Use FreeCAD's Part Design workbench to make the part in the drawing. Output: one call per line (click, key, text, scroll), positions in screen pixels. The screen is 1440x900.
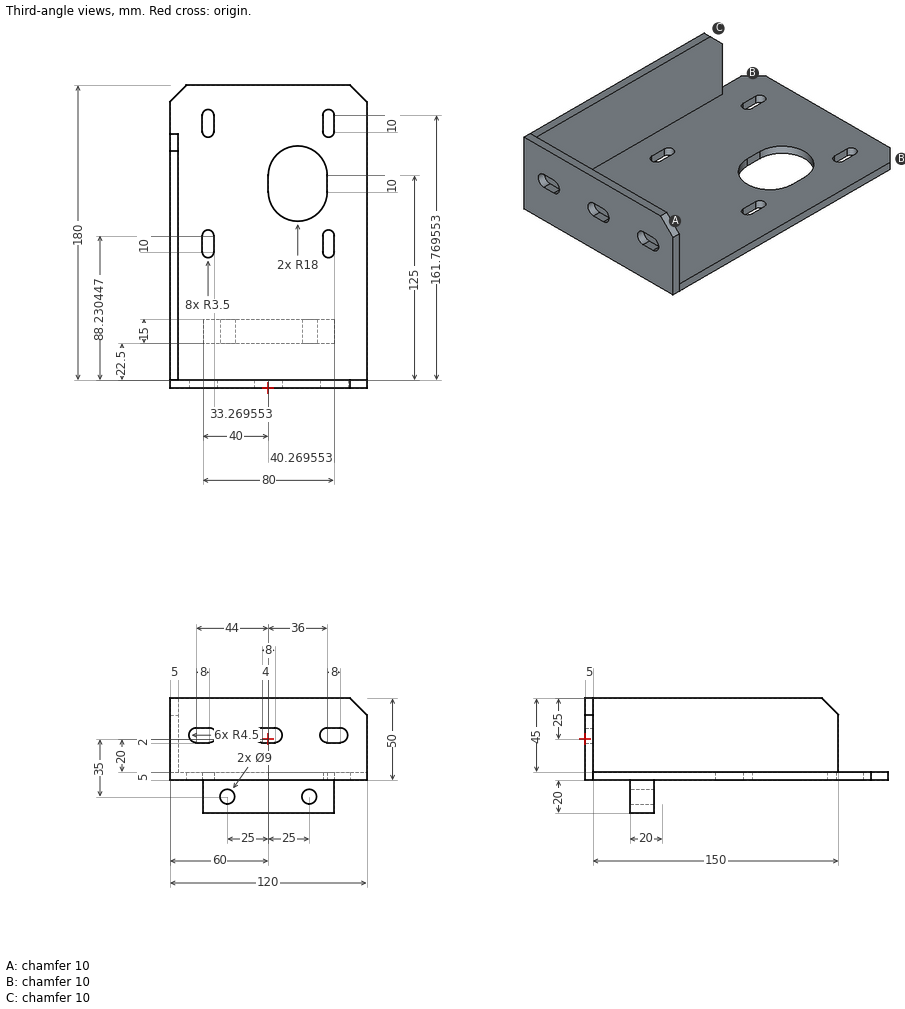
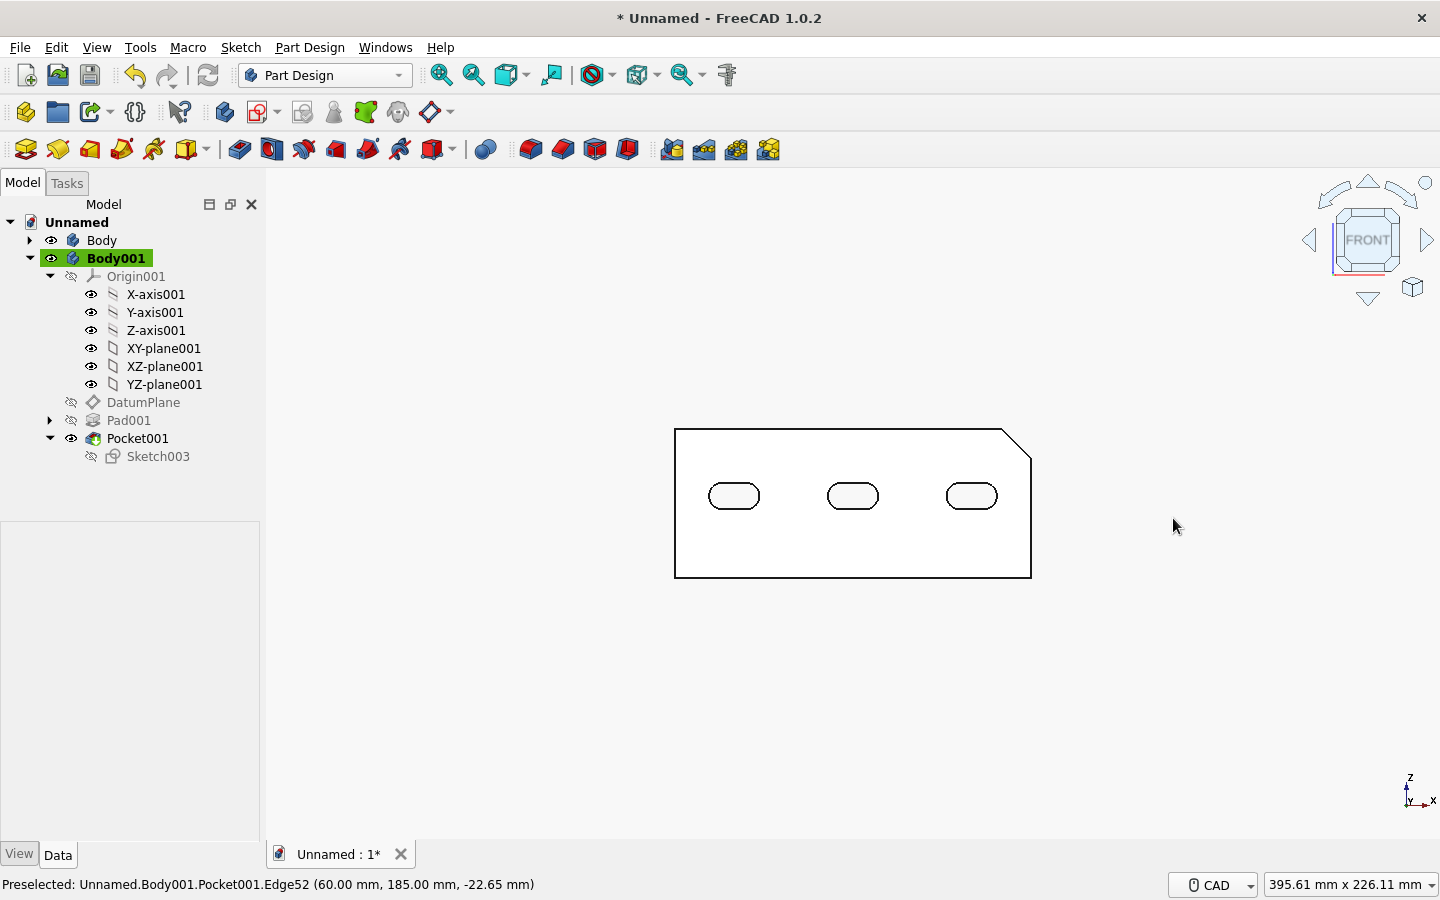
key(v)
key(f)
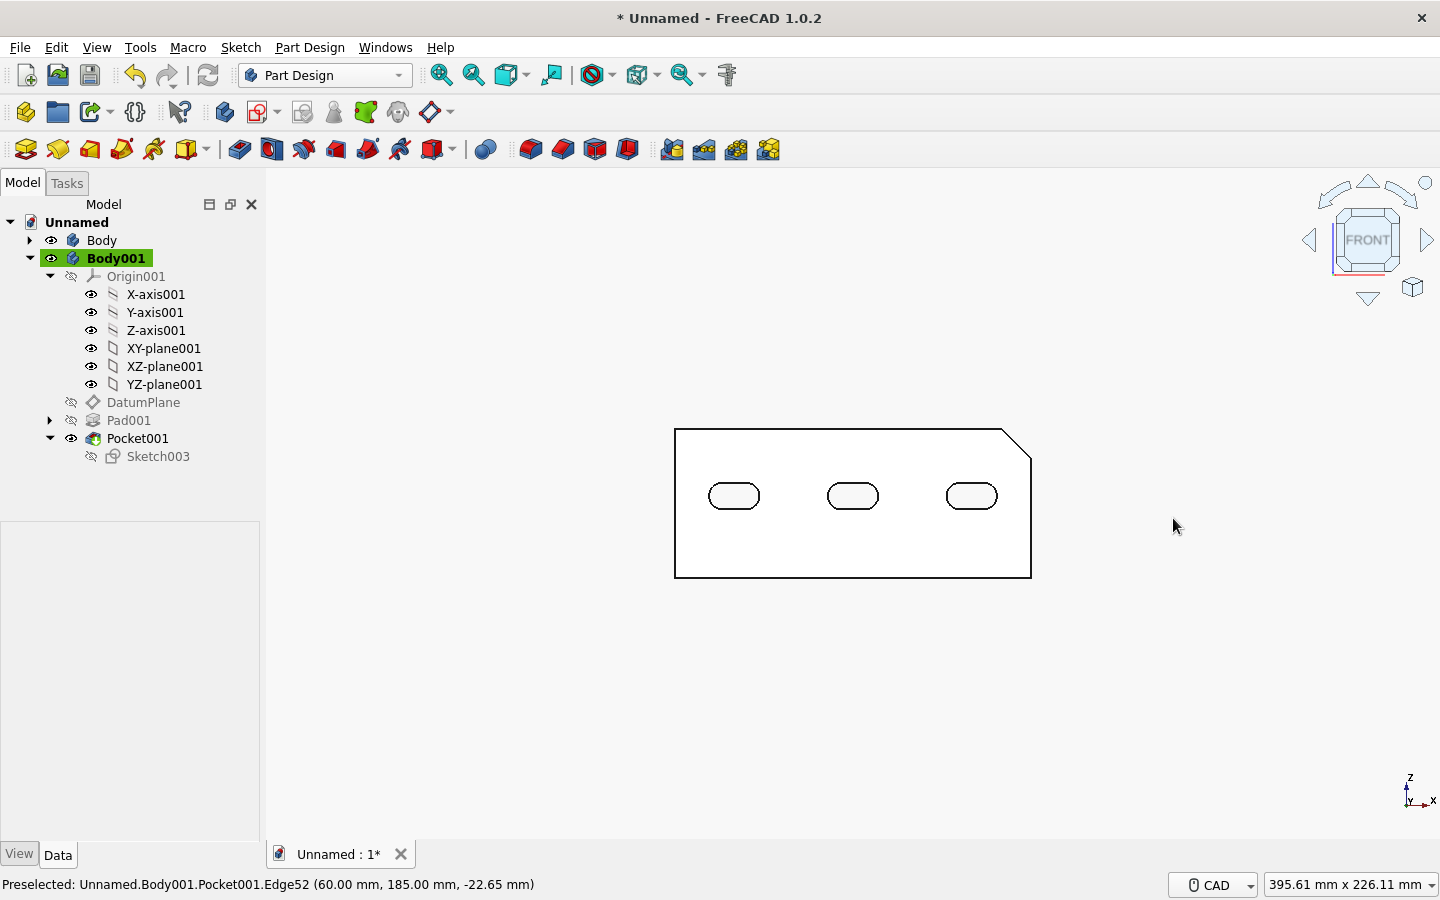
scroll(1031, 569, up, 5)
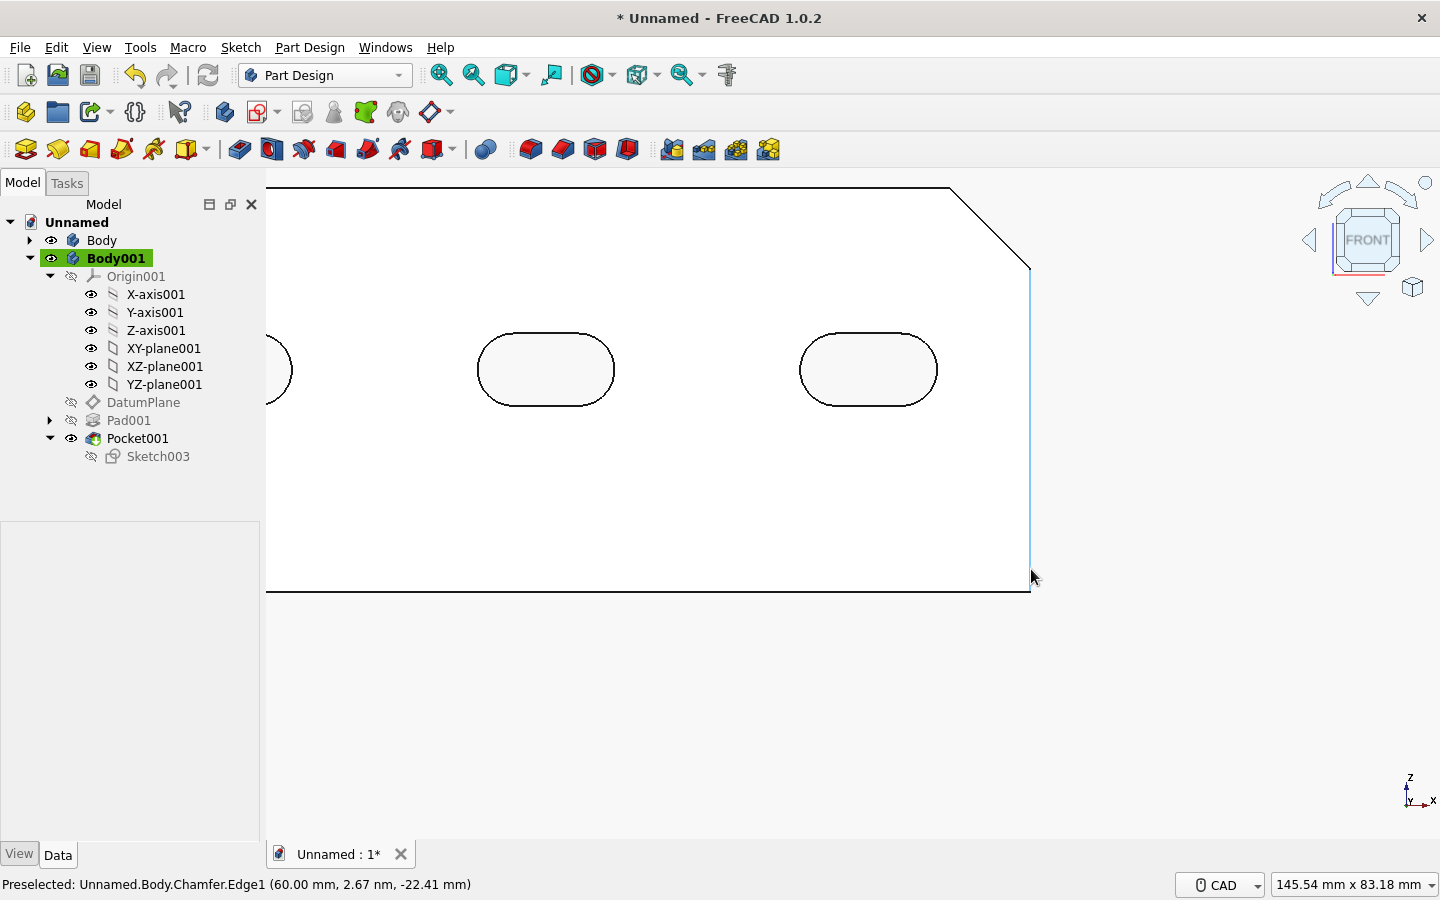
key(v)
key(f)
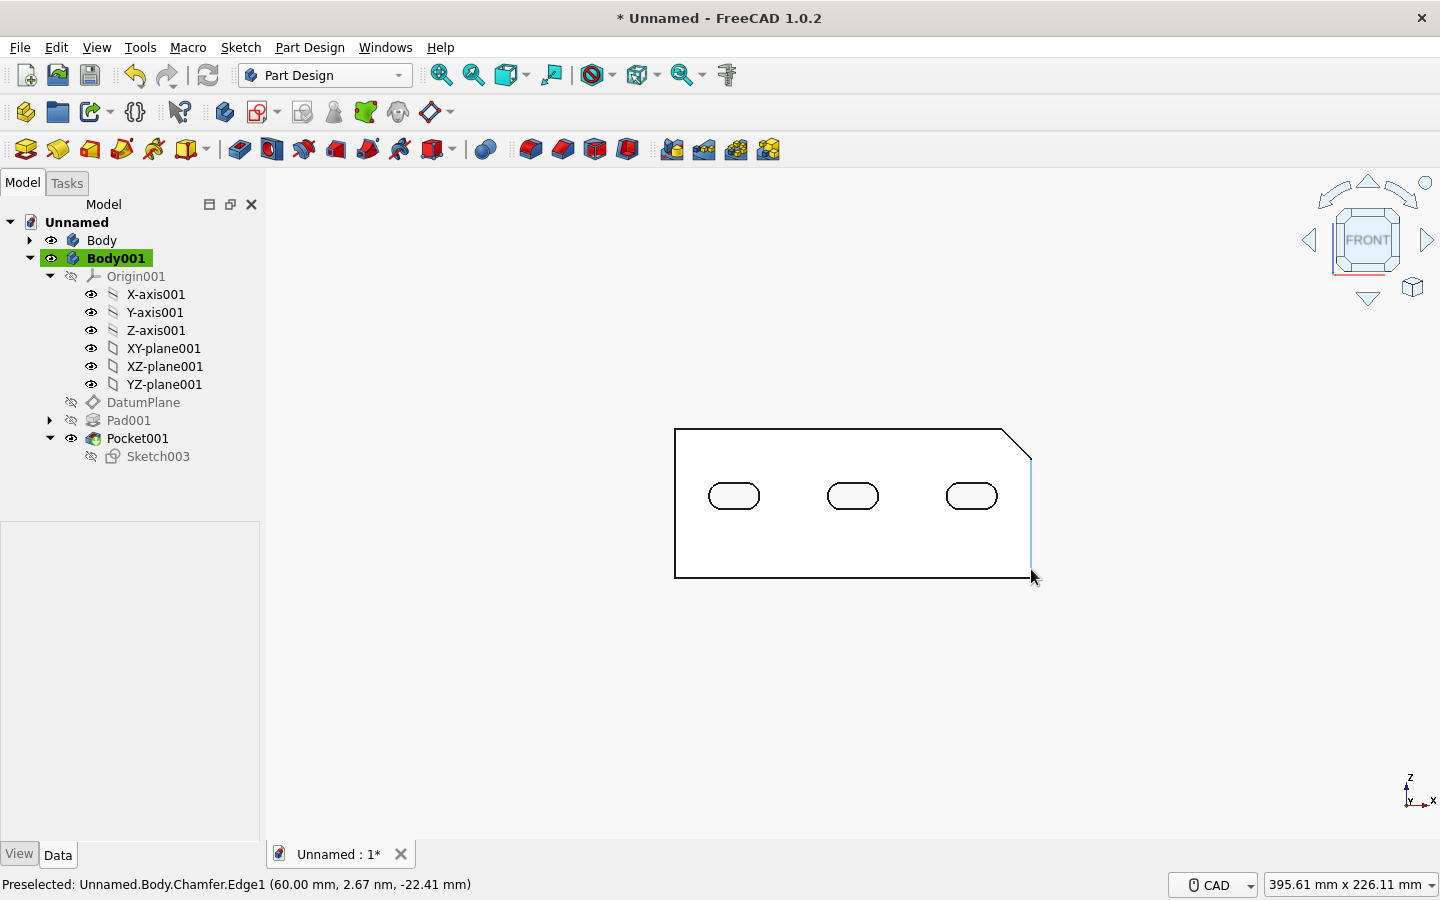
key(3)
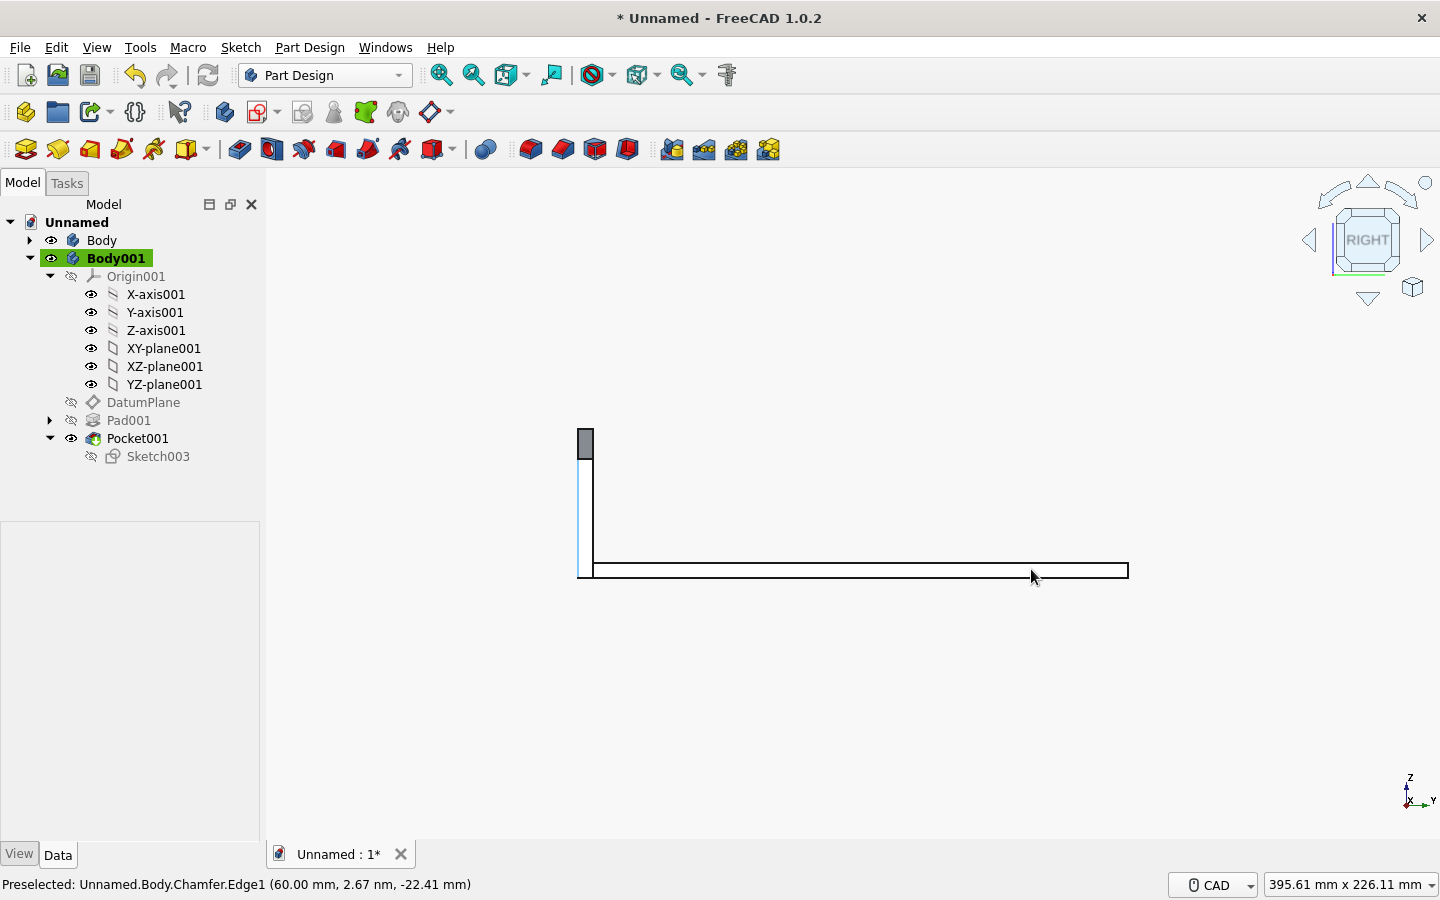
click(1128, 569)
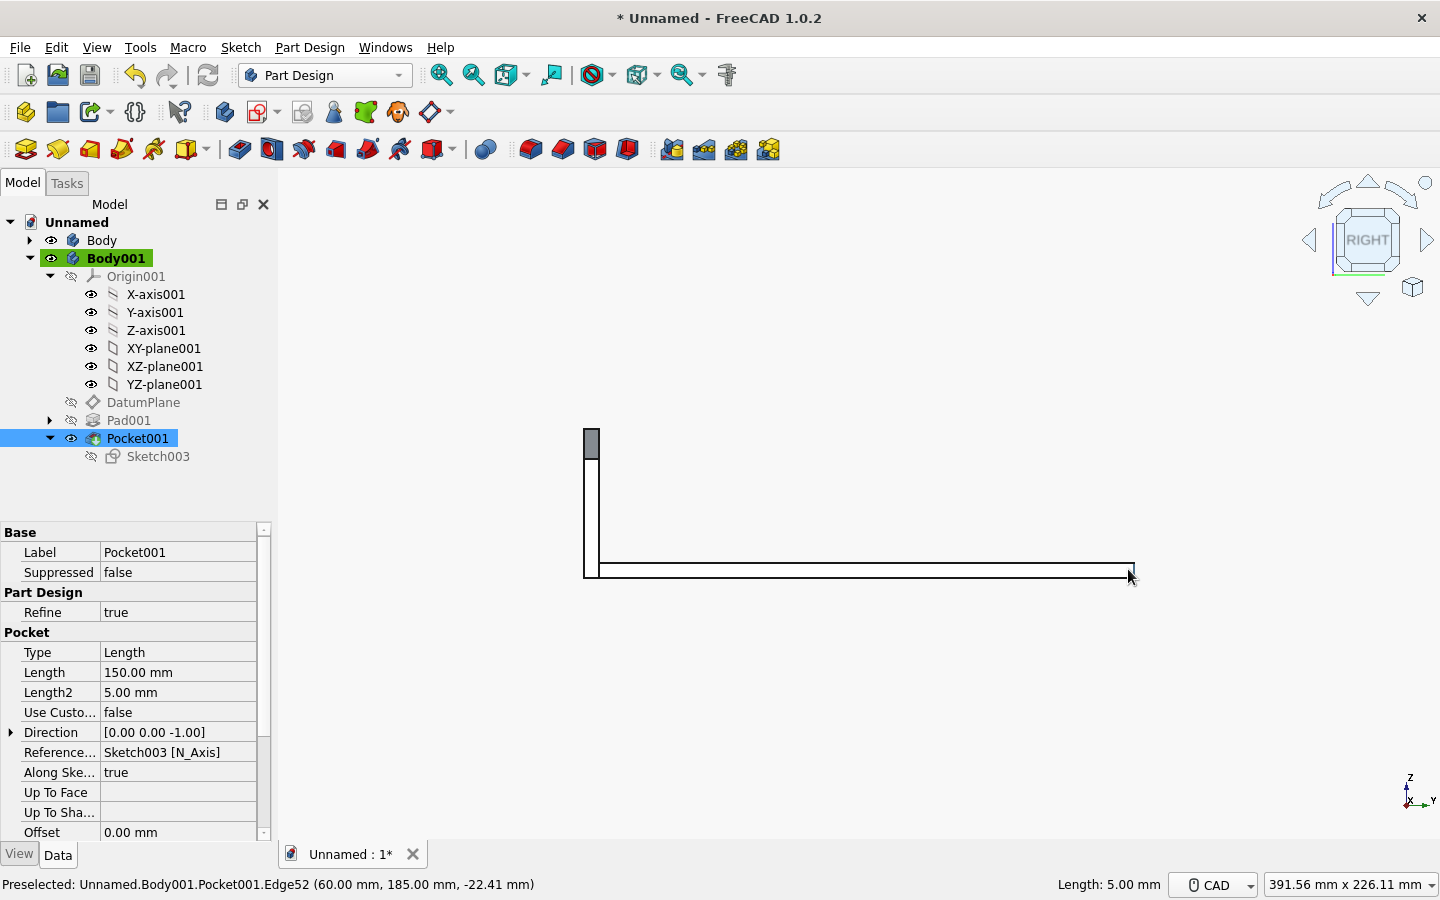
scroll(1134, 569, up, 5)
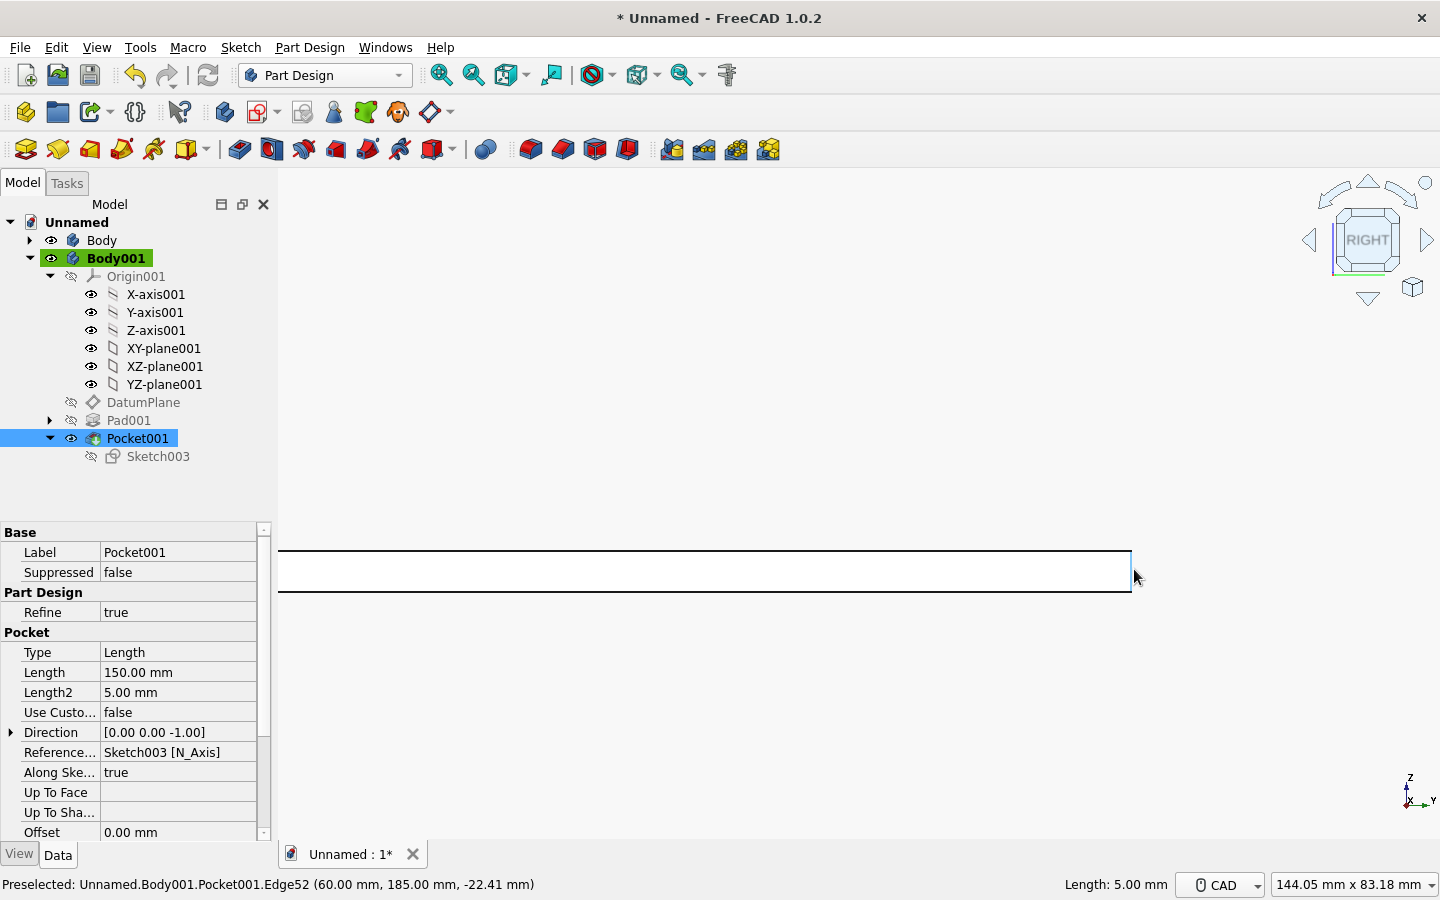
click(442, 76)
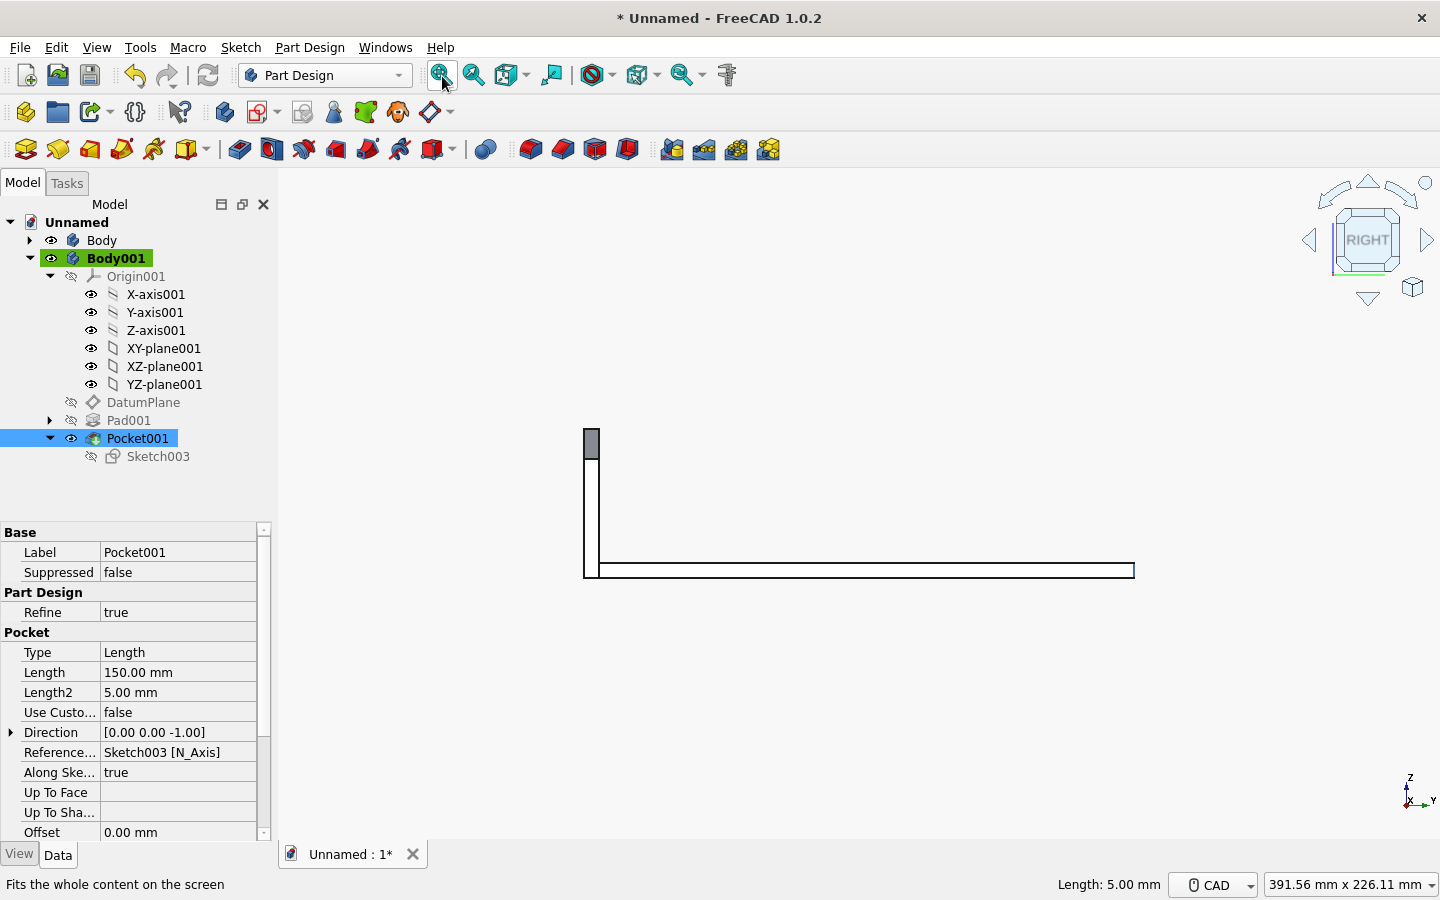
key(5)